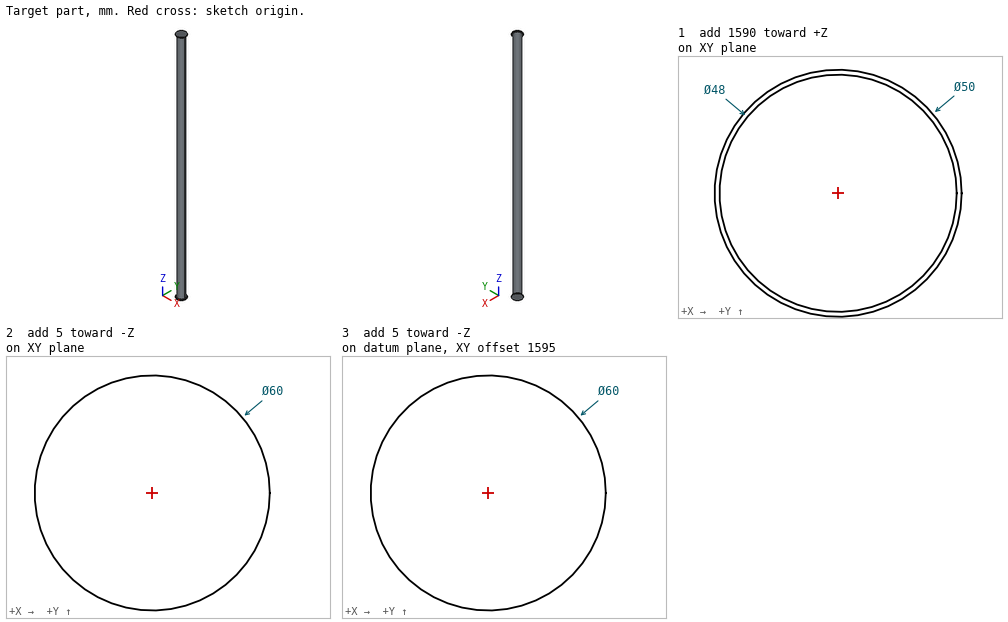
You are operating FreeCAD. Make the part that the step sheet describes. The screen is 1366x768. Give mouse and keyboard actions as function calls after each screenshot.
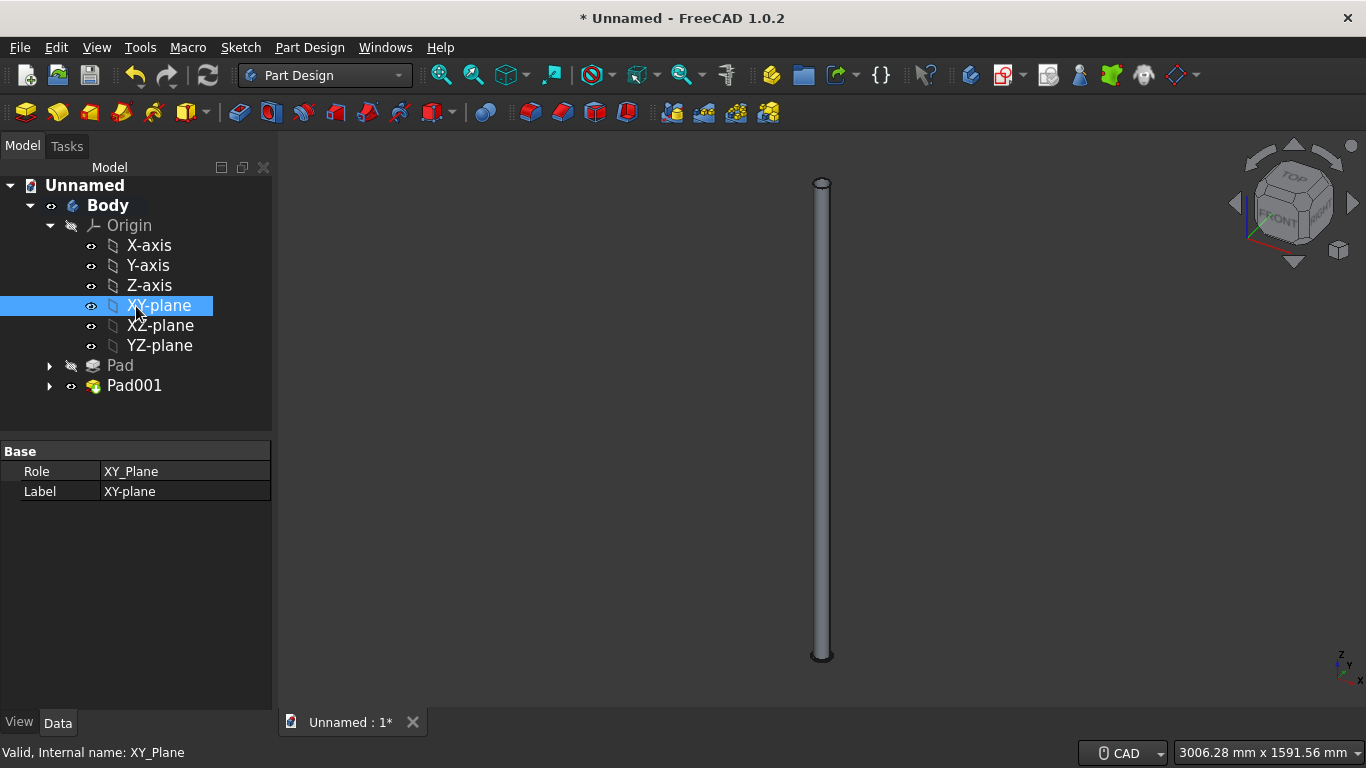
click(1176, 76)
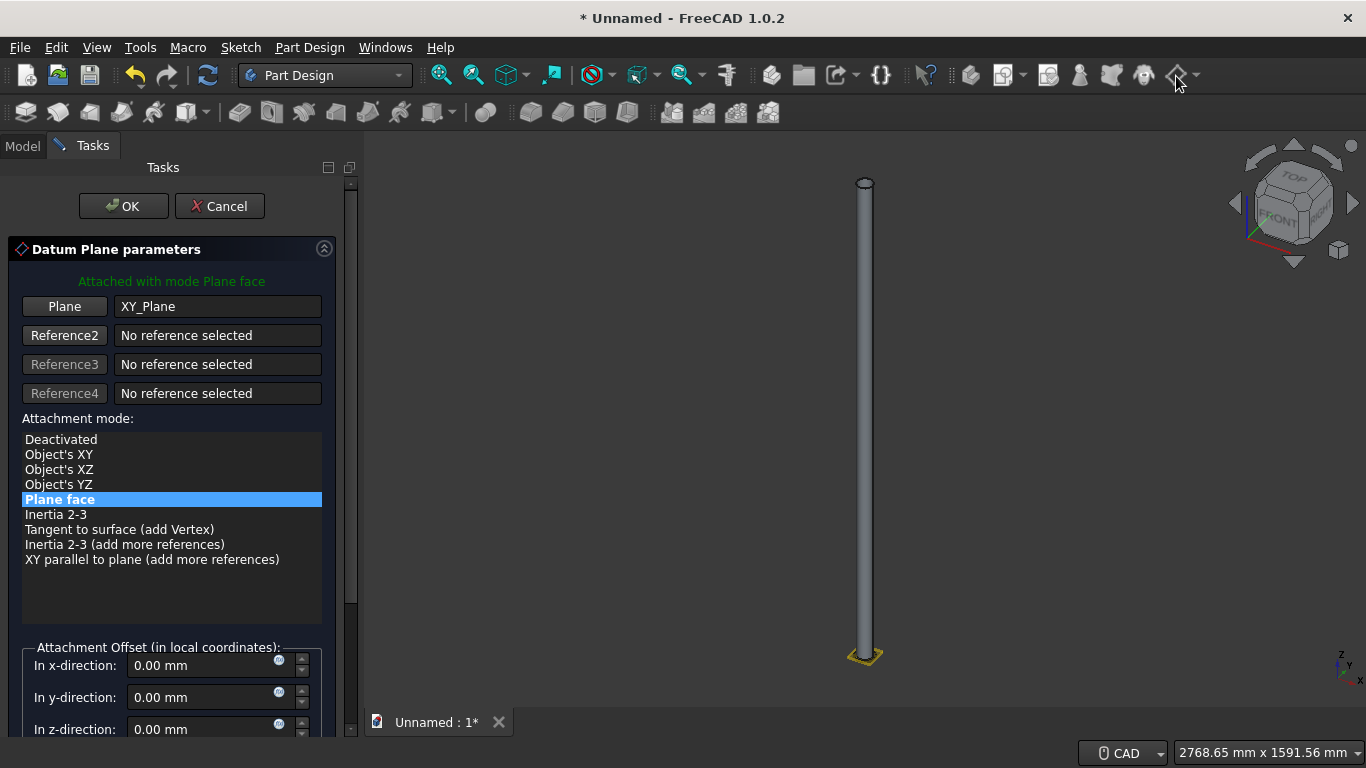
scroll(351, 456, down, 2)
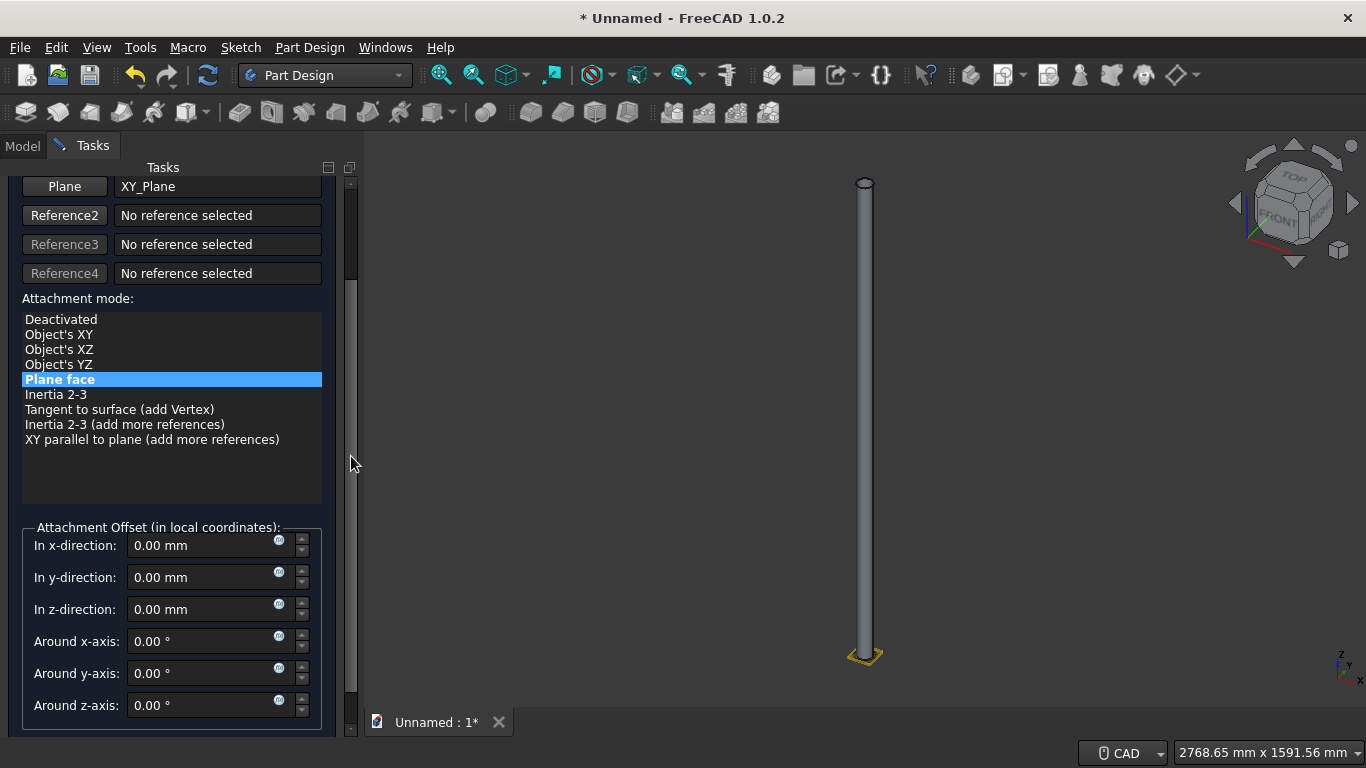
triple_click(210, 609)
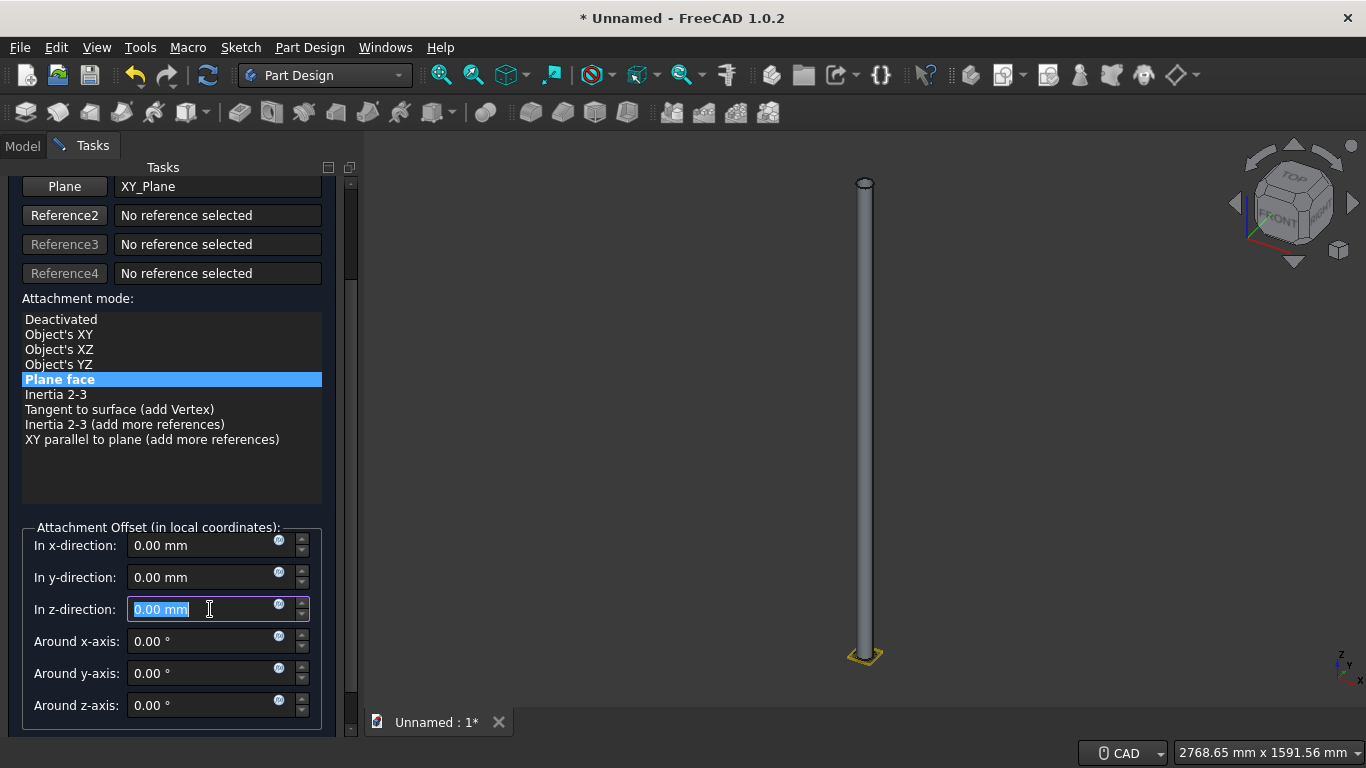
text(1595)
key(Tab)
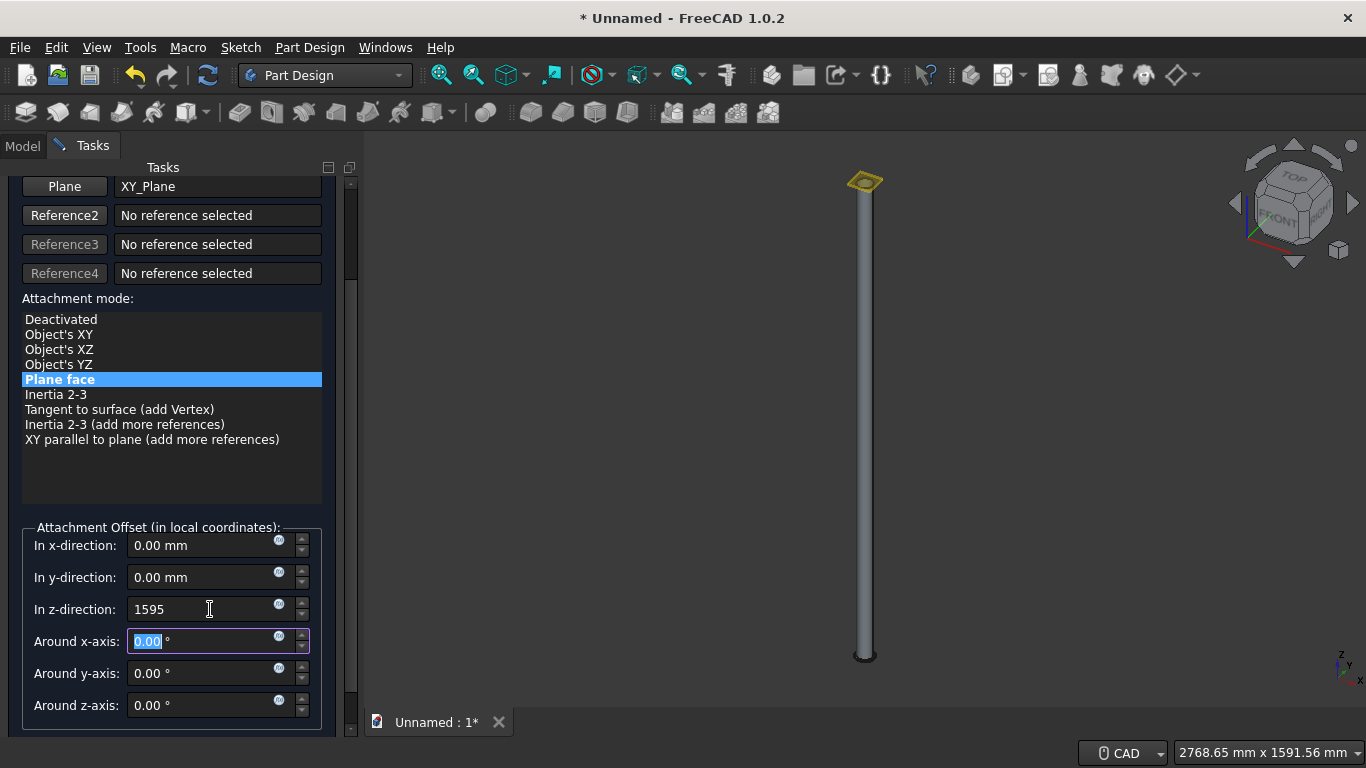
scroll(351, 456, up, 3)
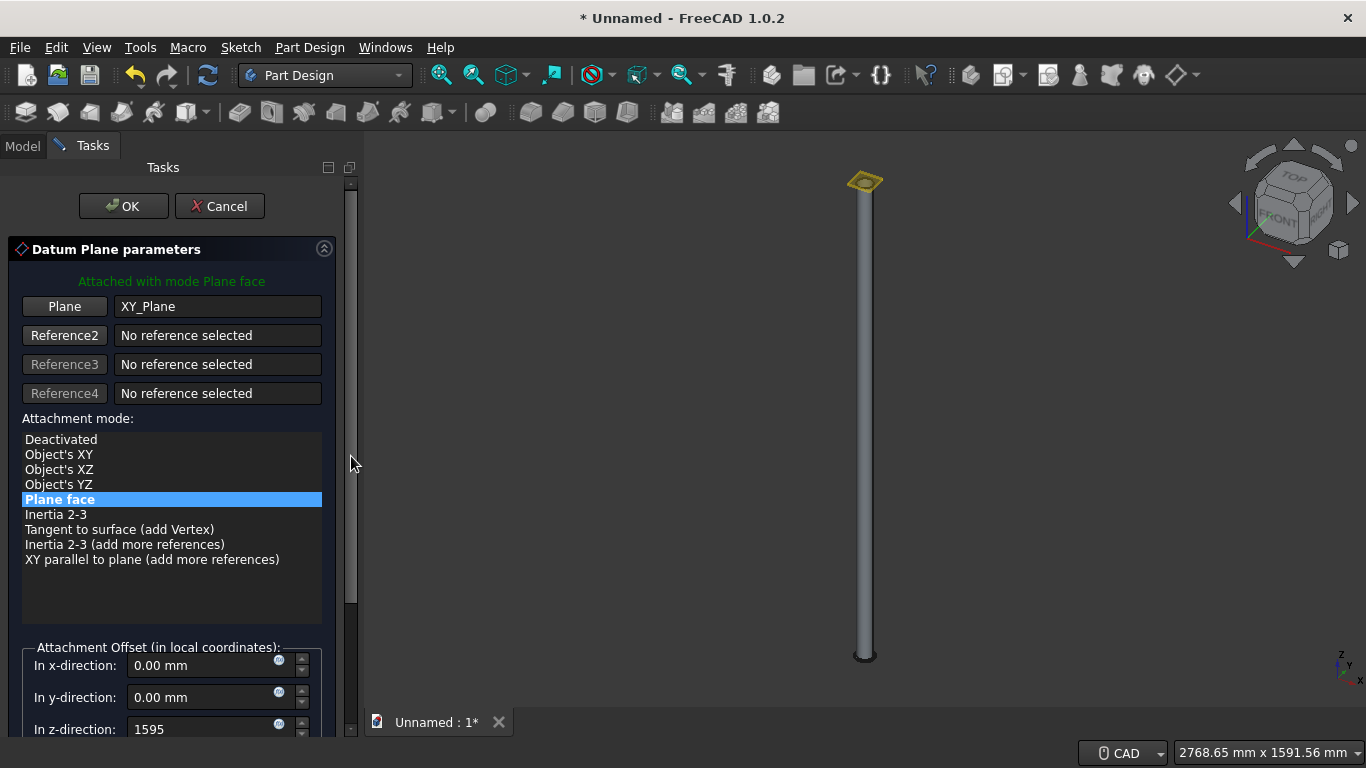
click(124, 206)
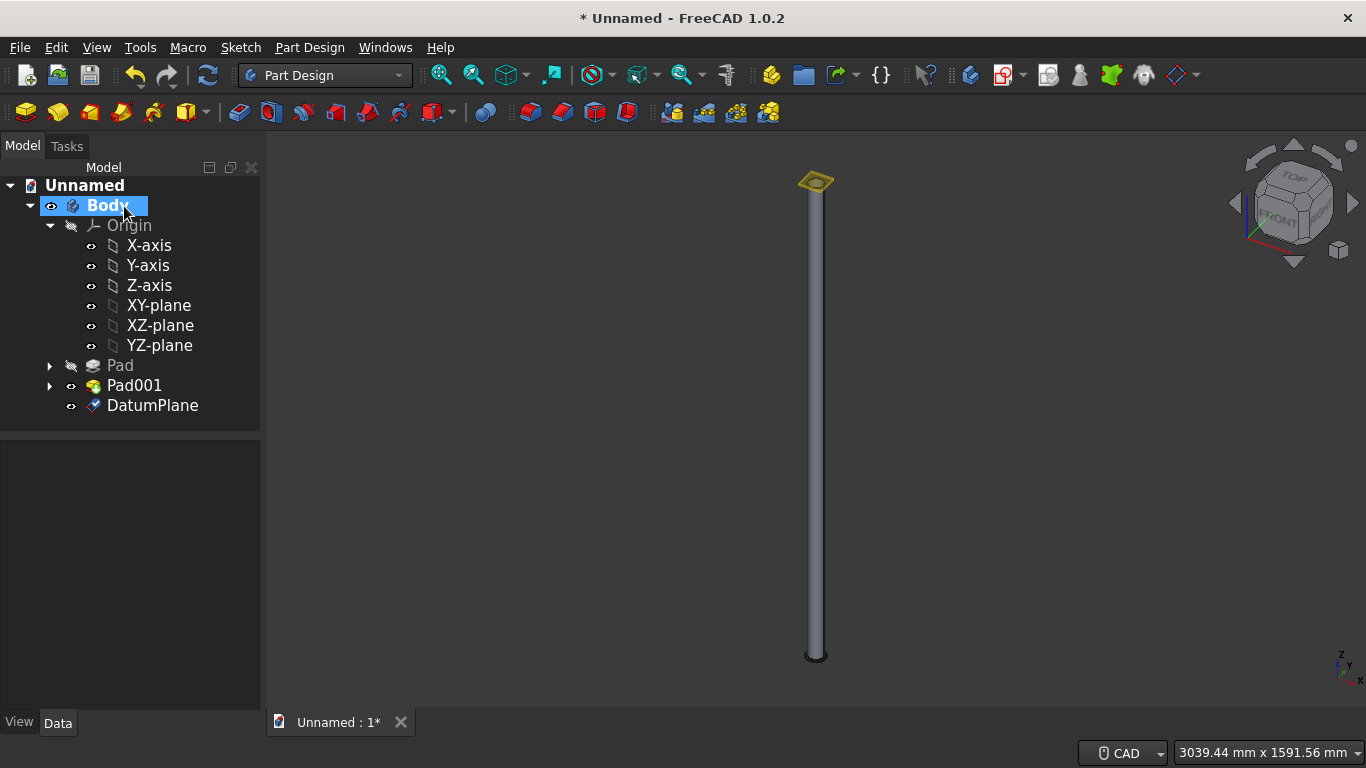
click(116, 406)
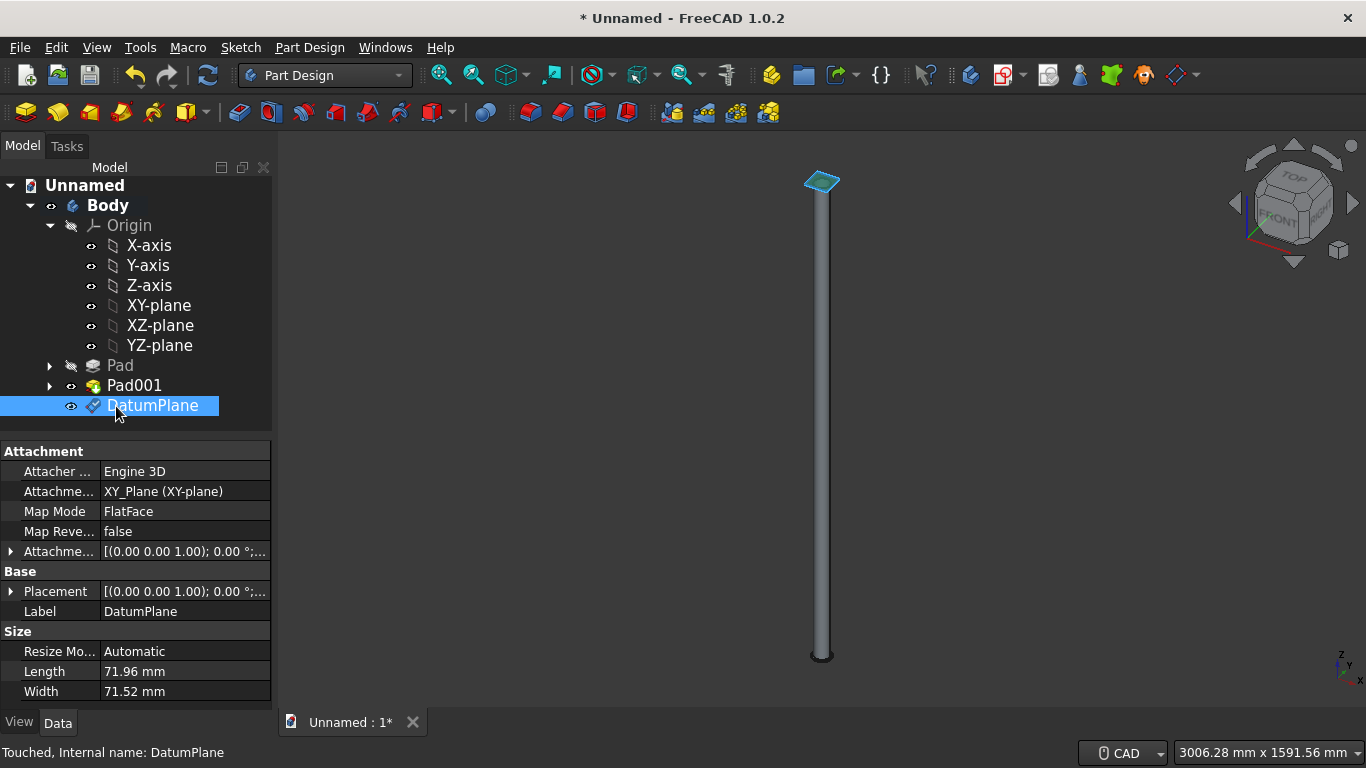
click(1004, 76)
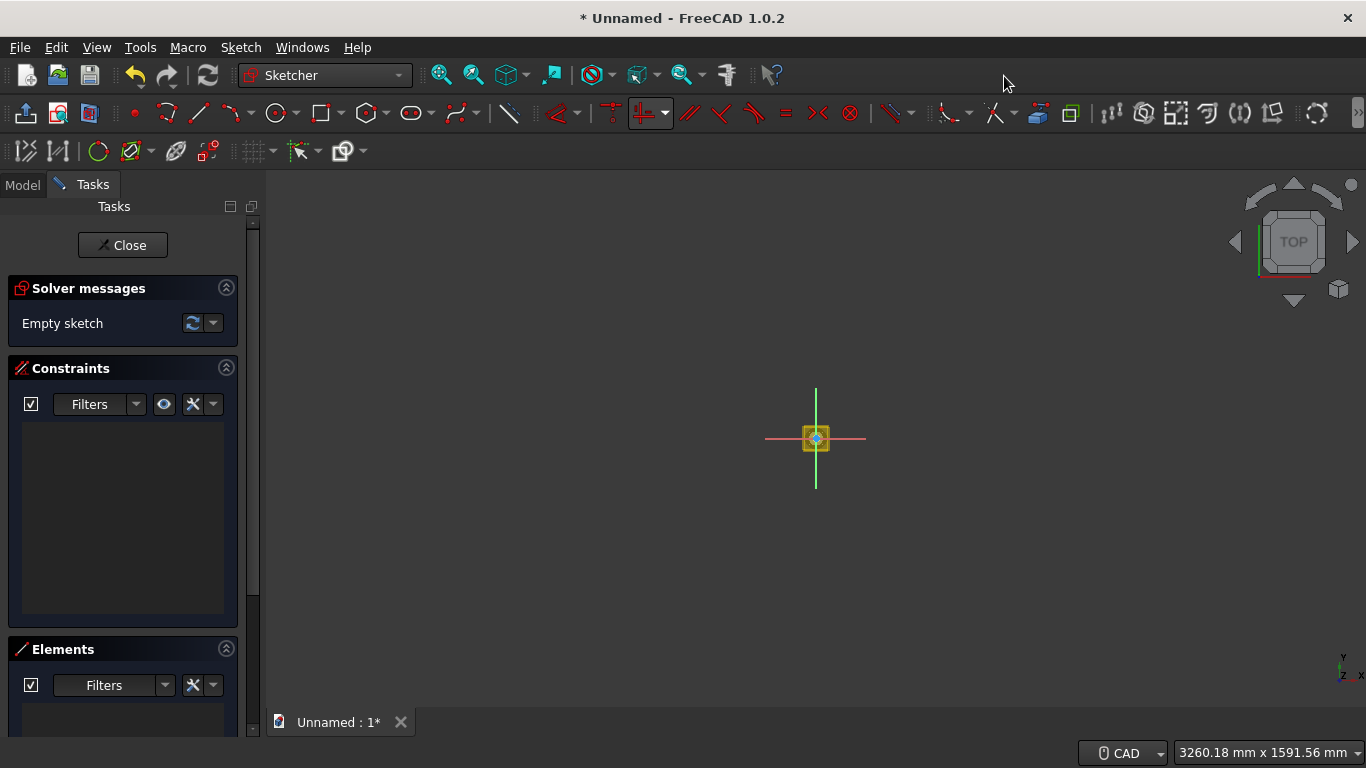
scroll(820, 439, up, 14)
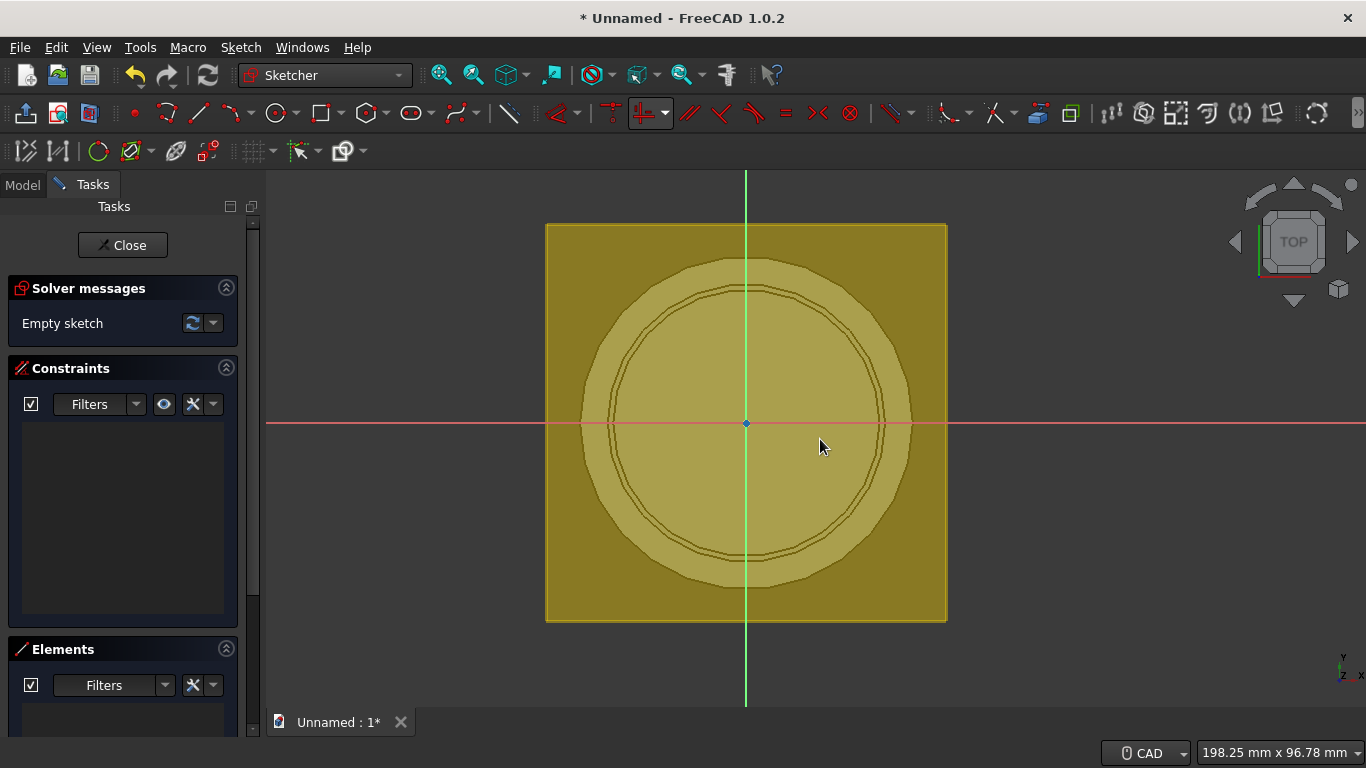
click(276, 114)